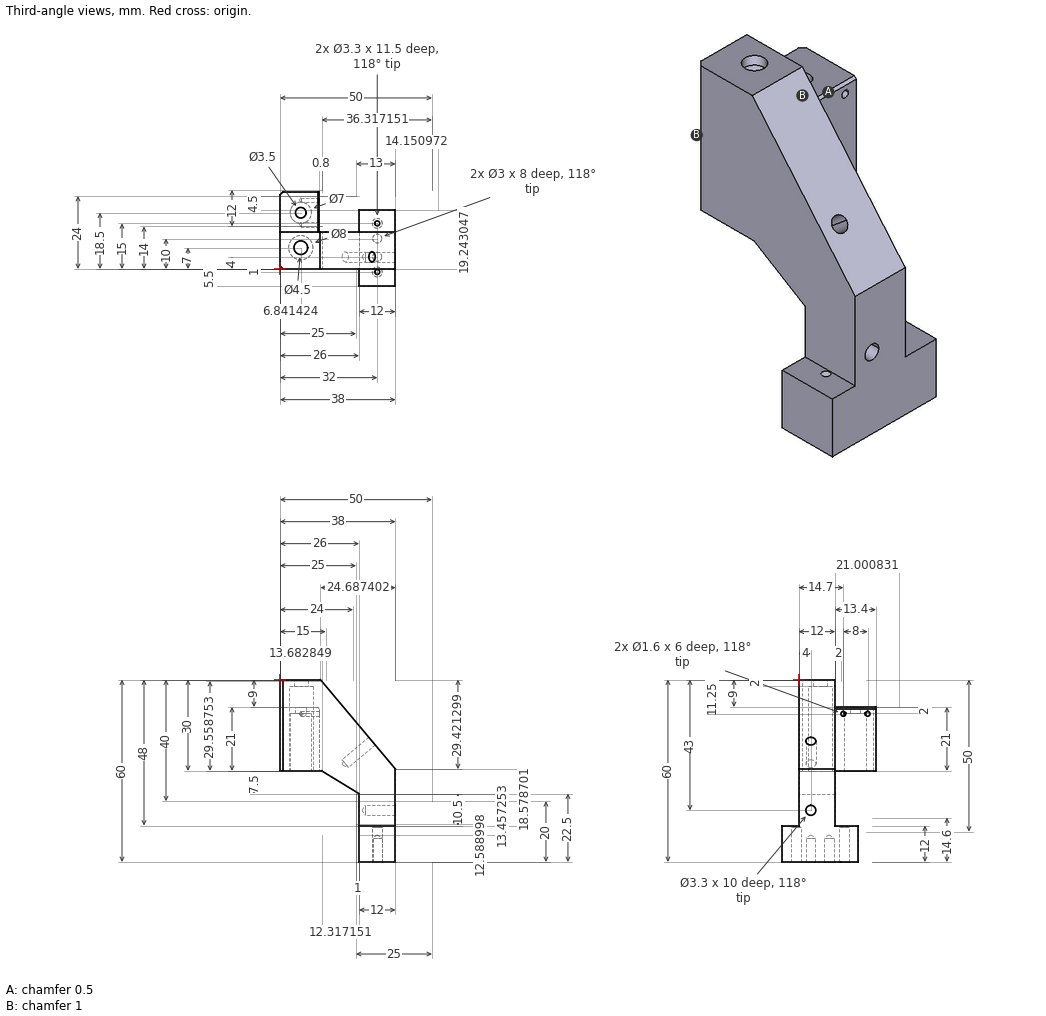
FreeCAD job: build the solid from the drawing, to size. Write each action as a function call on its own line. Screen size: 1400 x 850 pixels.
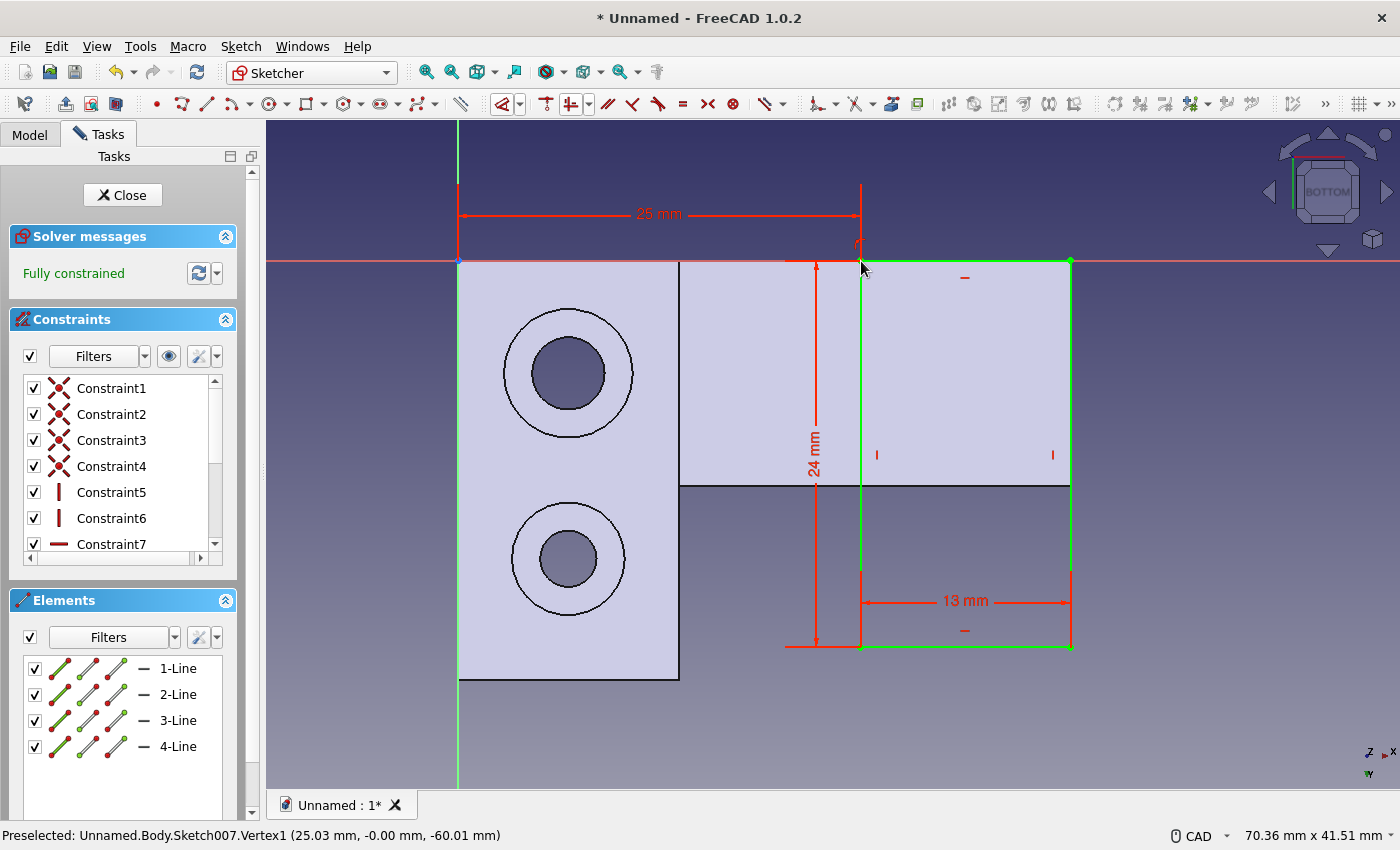
click(123, 195)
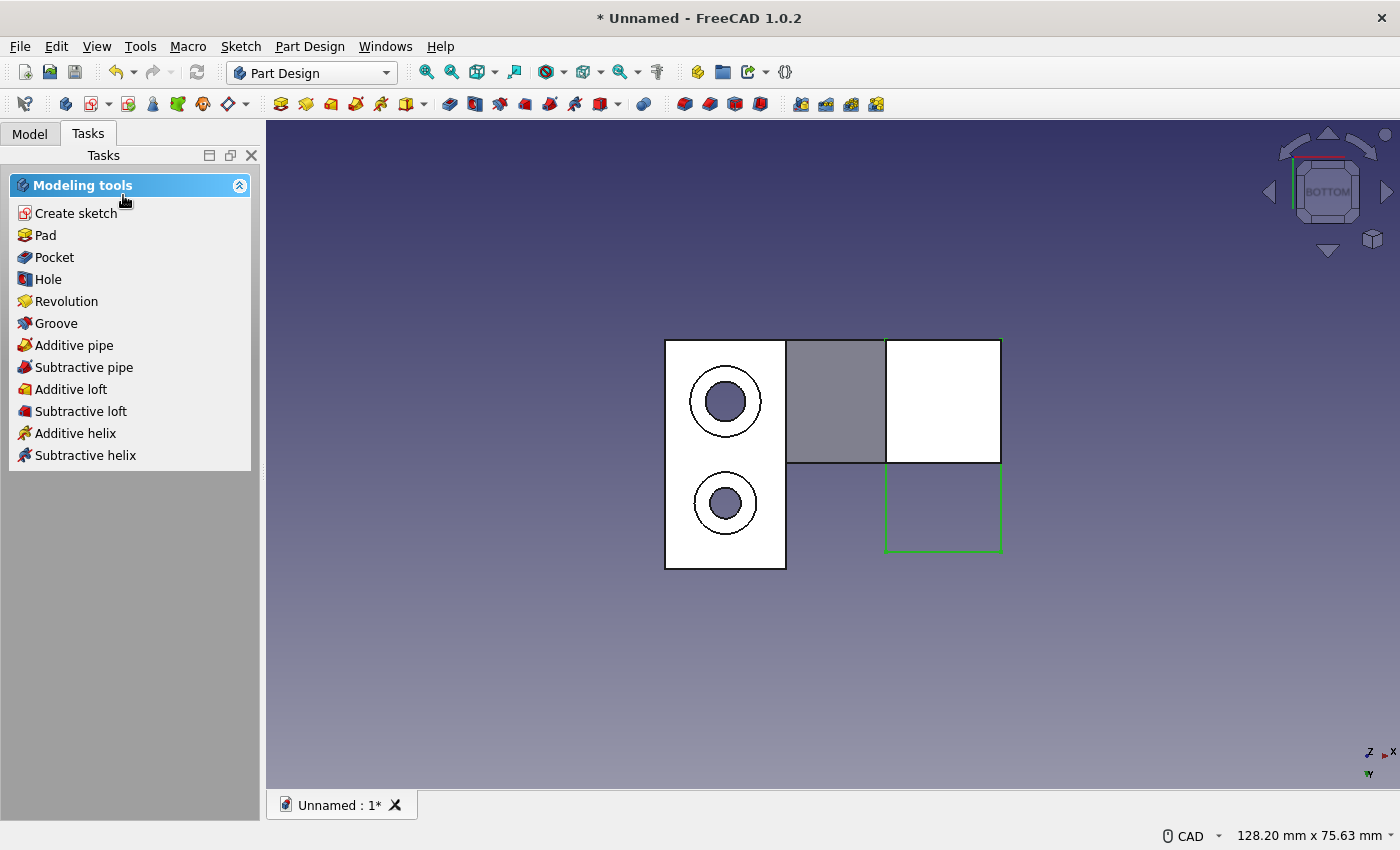
click(281, 104)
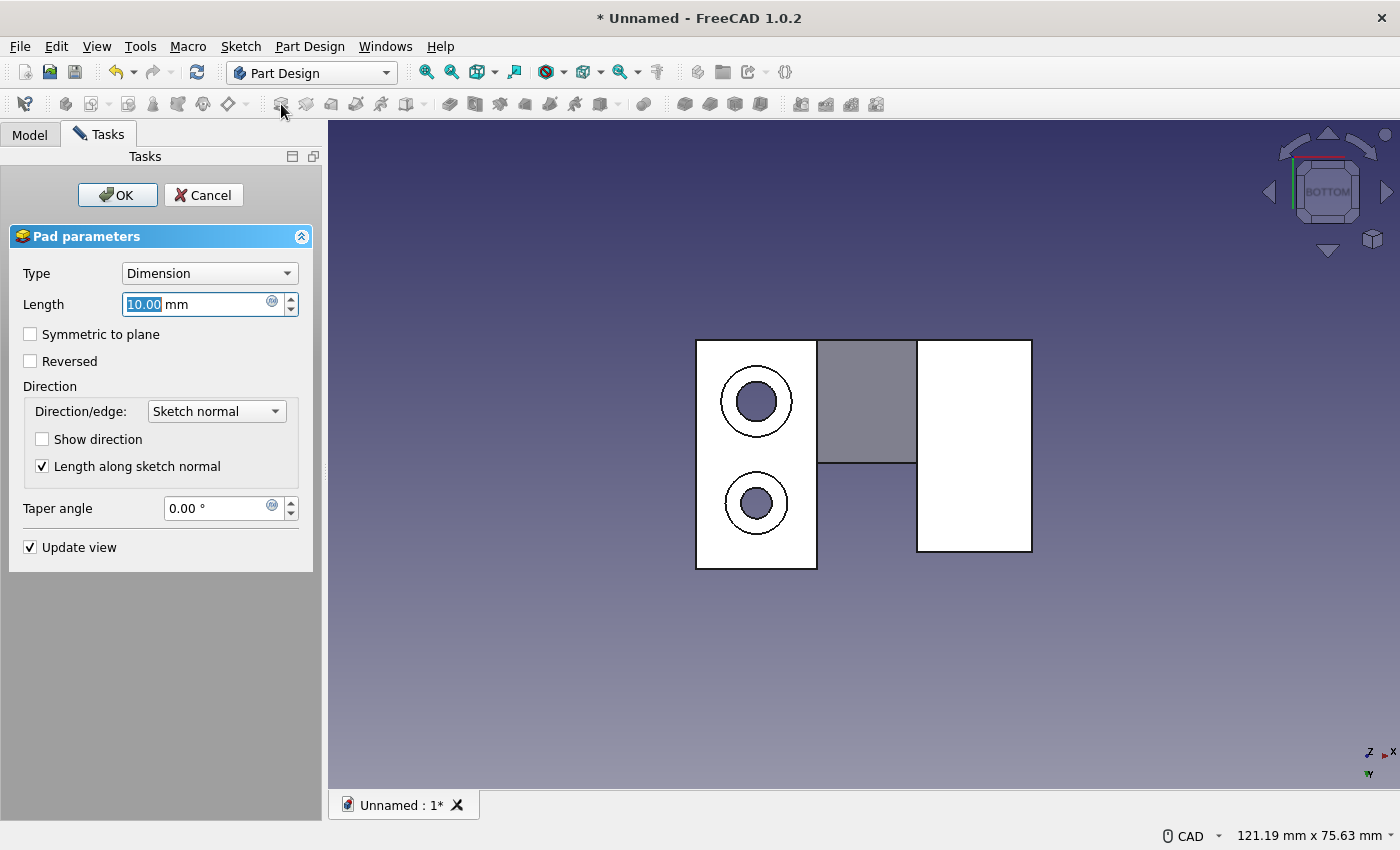
text(12)
key(Tab)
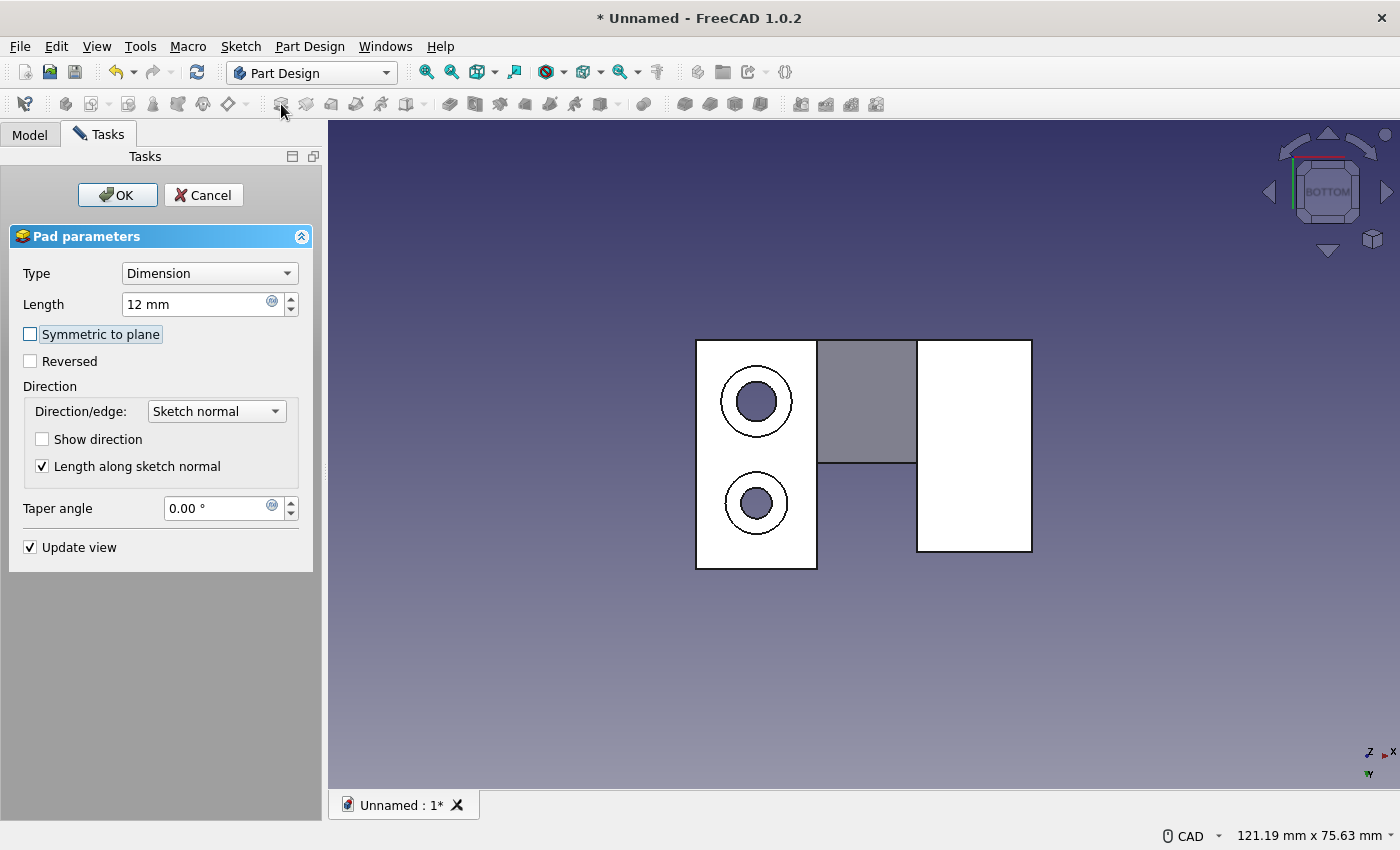
click(31, 361)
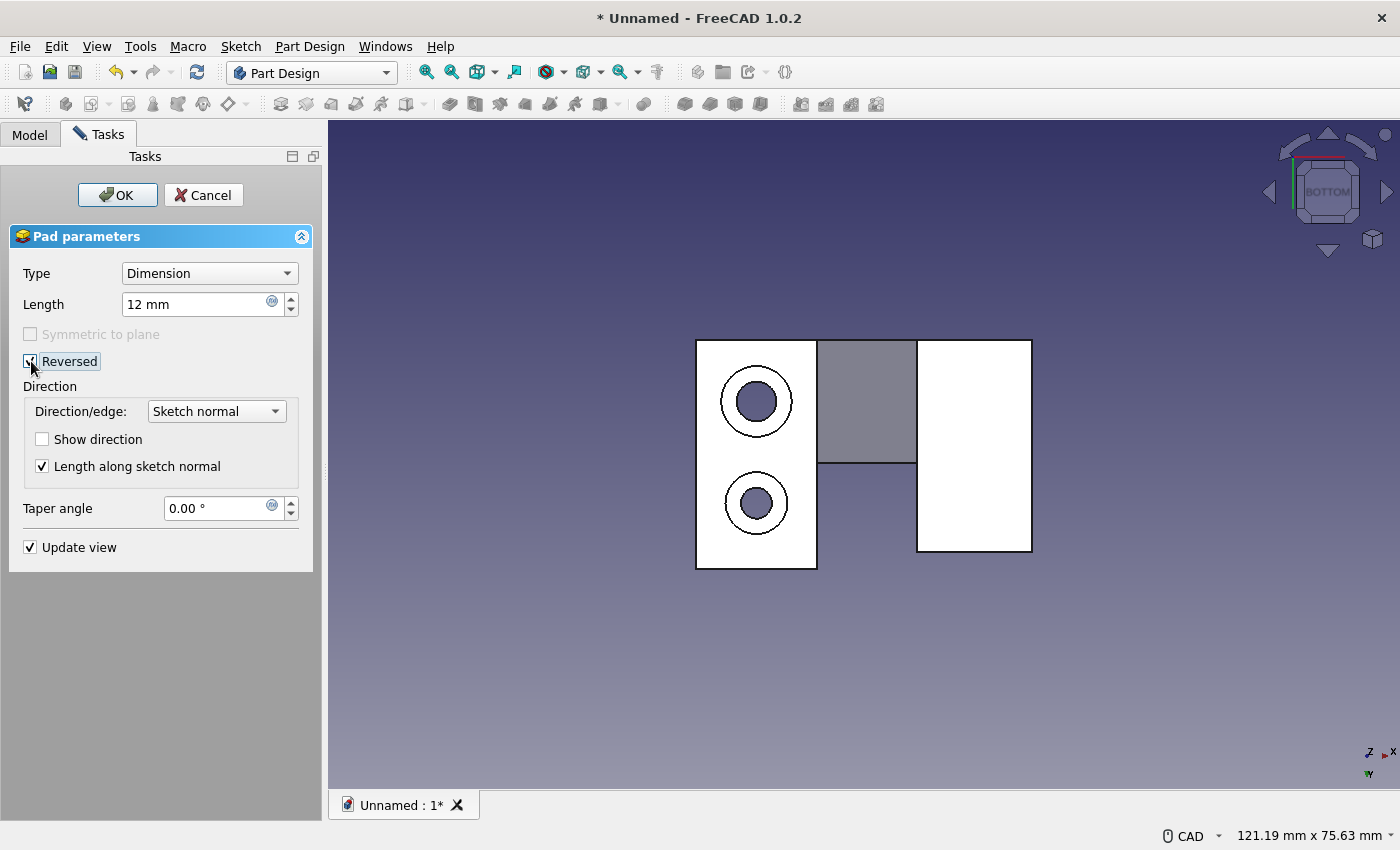
click(118, 195)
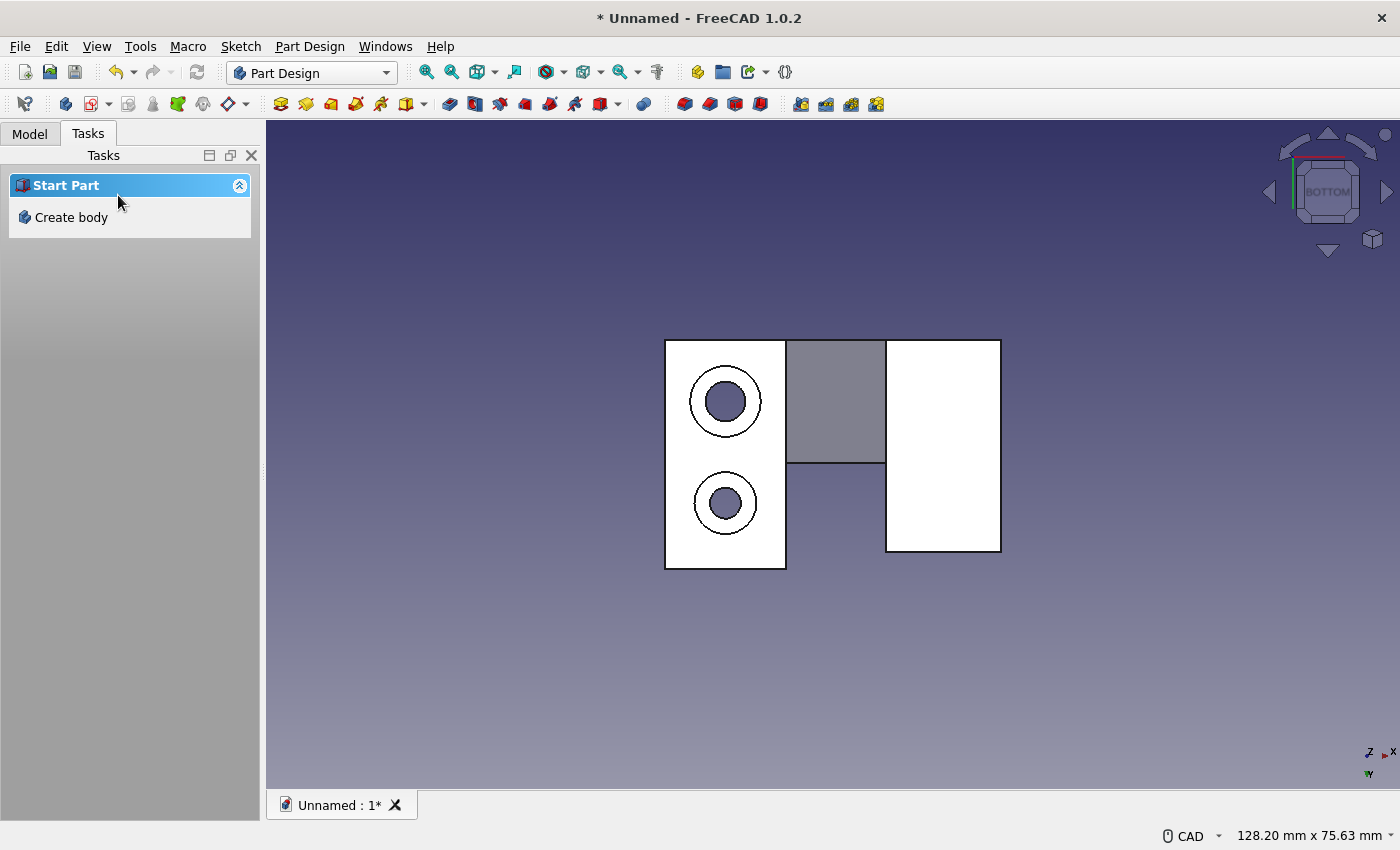
click(427, 72)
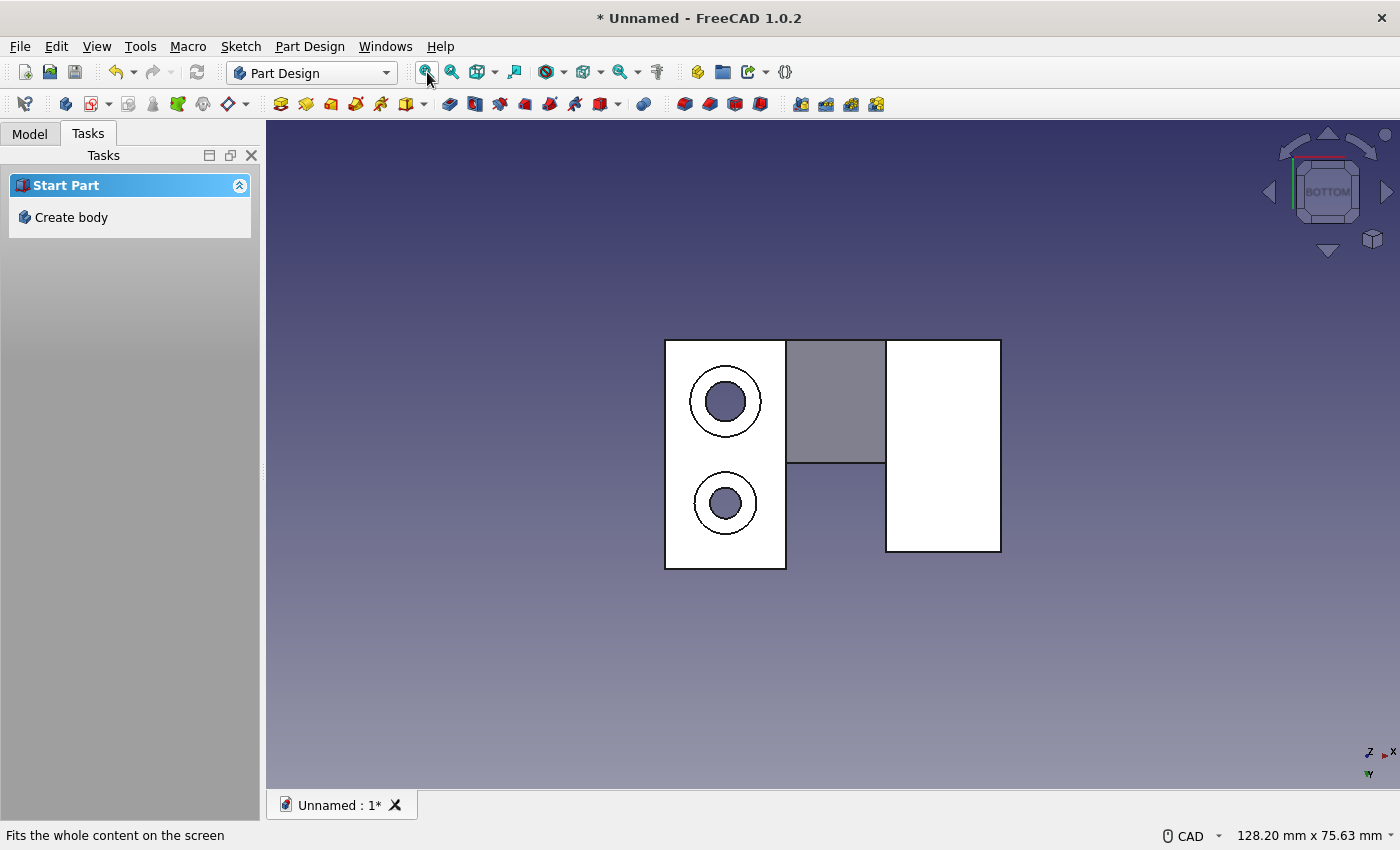
key(4)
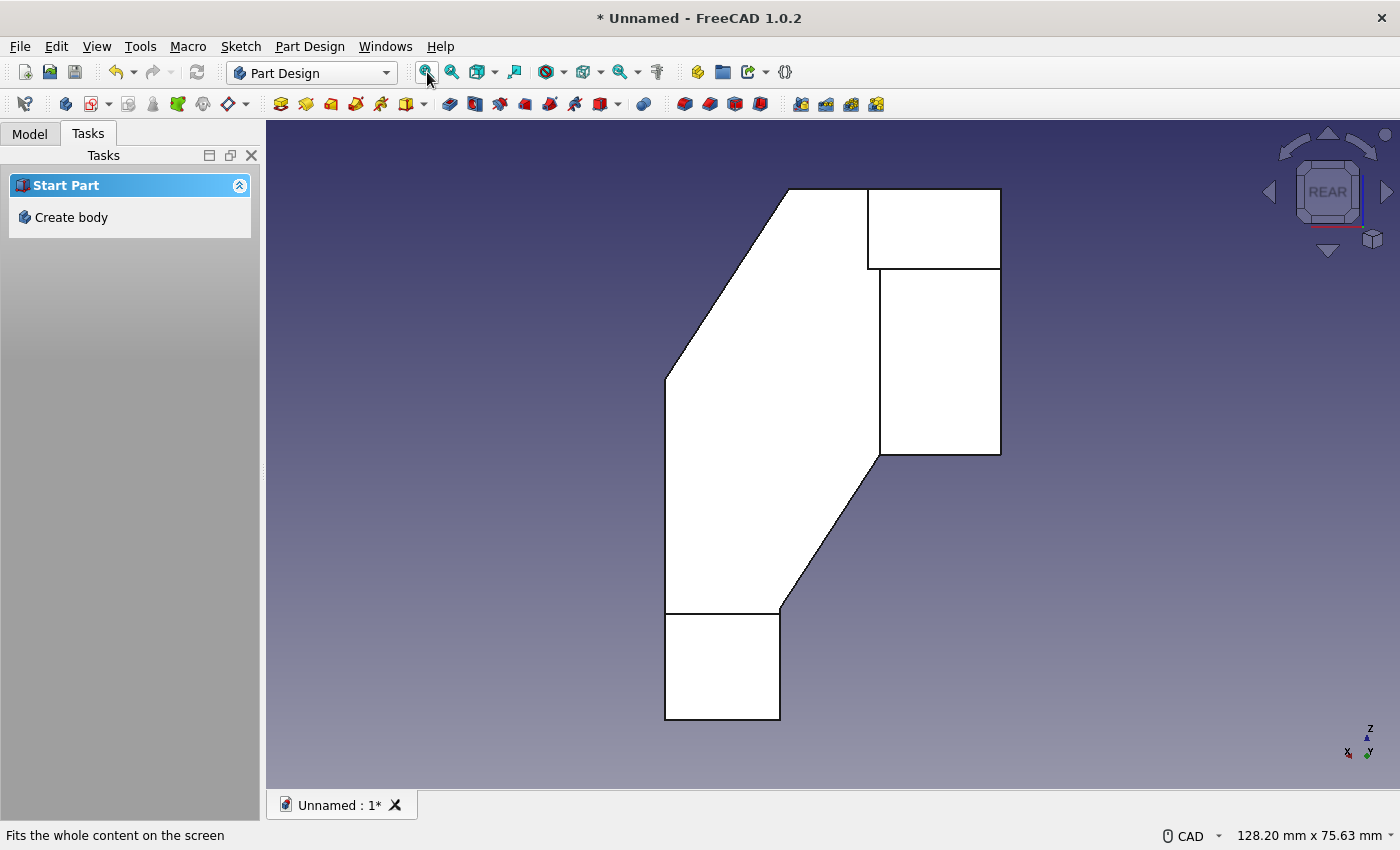
click(722, 666)